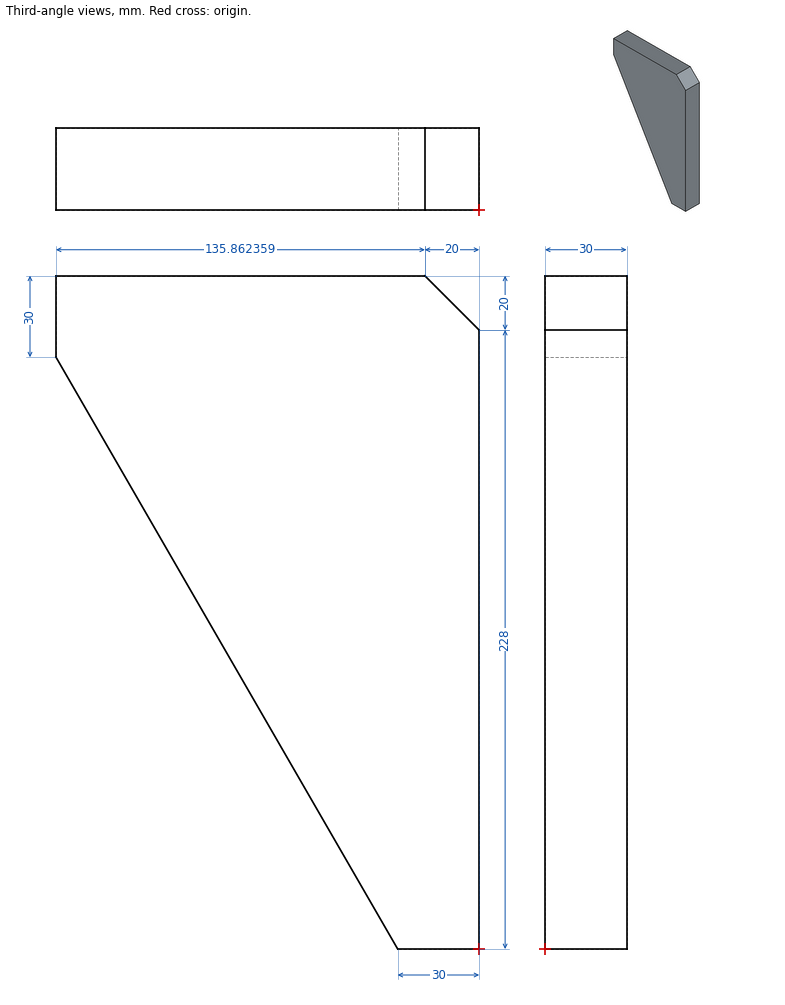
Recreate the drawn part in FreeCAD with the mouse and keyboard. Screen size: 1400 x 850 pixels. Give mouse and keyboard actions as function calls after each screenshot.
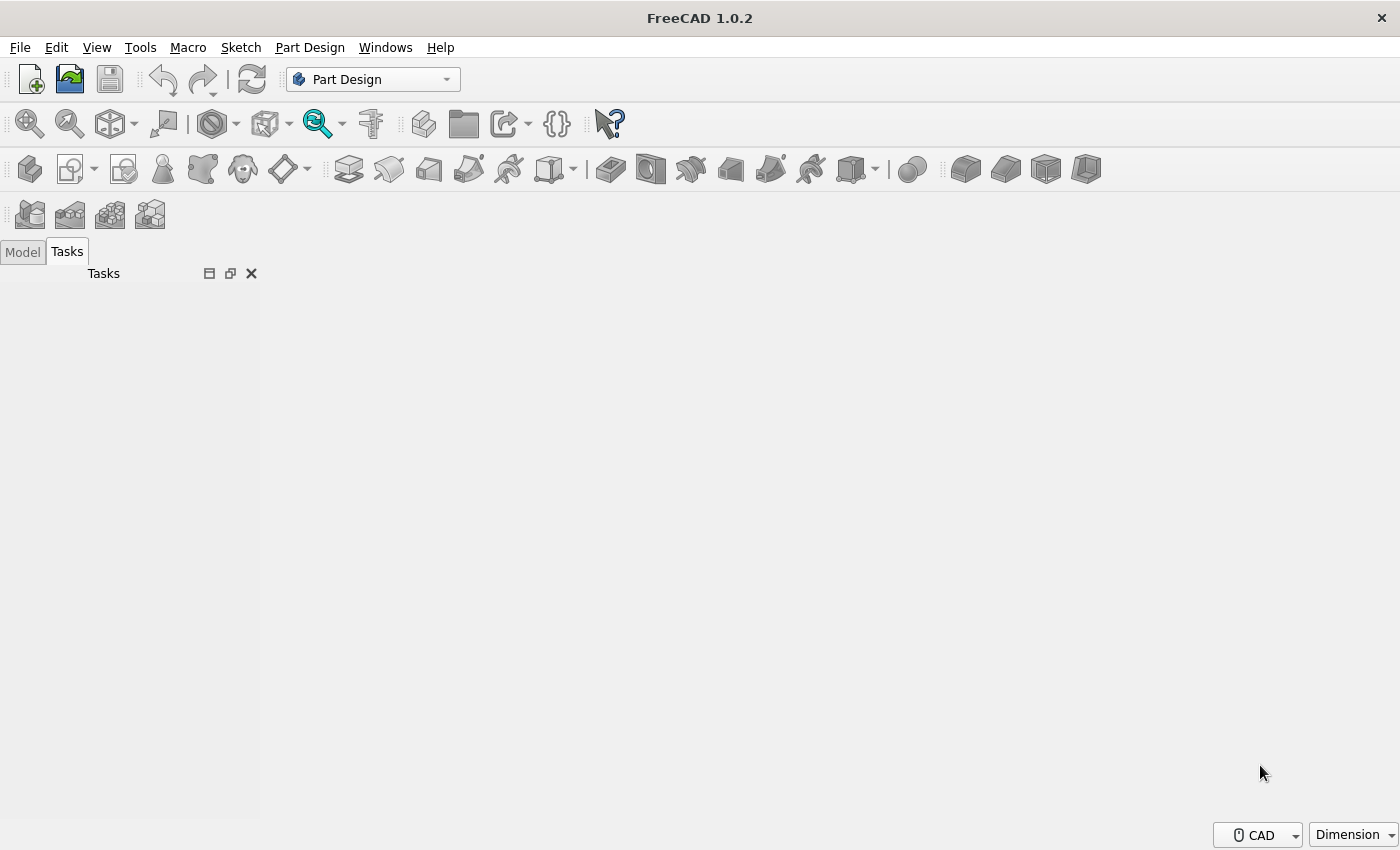
key(ctrl+n)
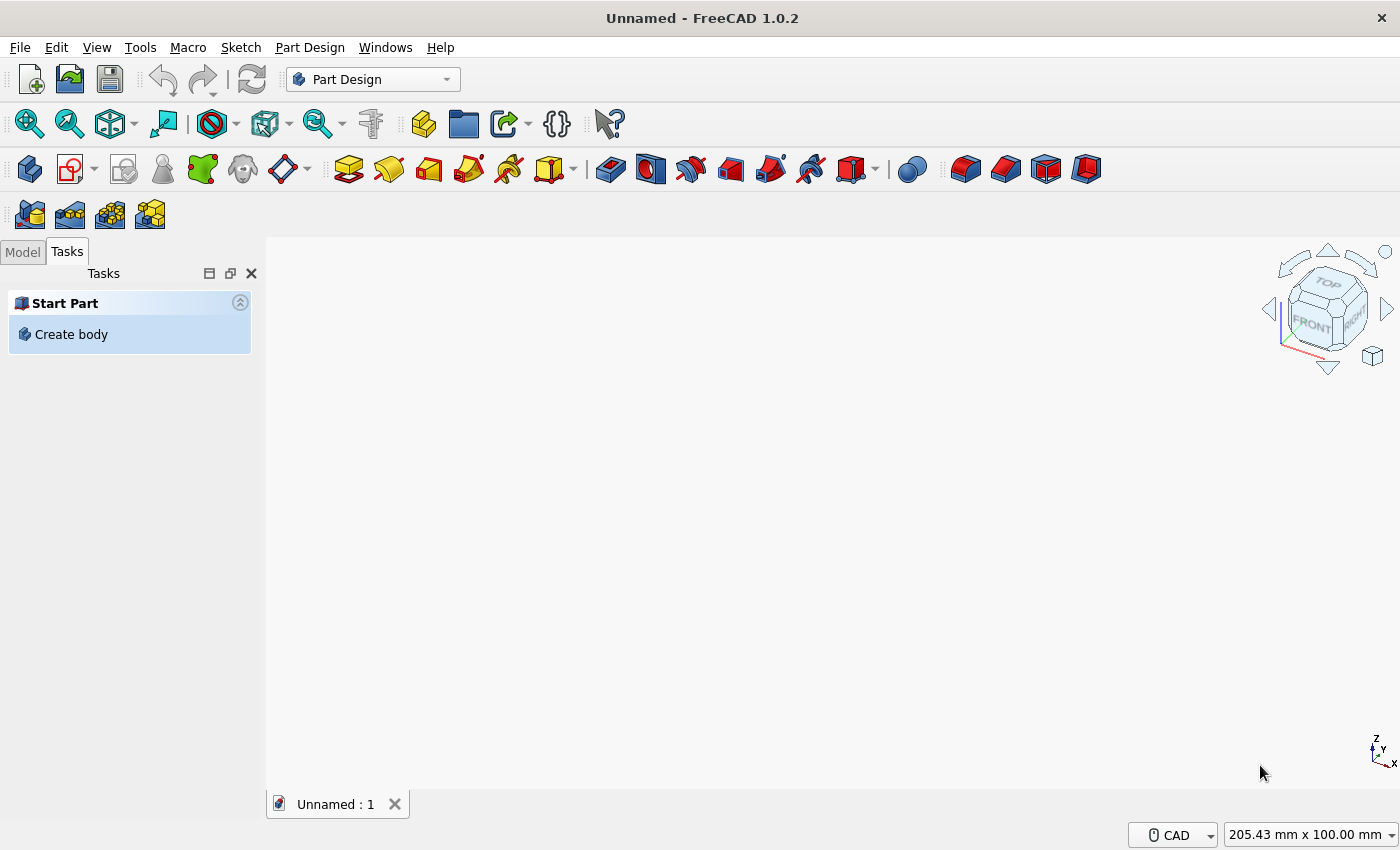
click(70, 170)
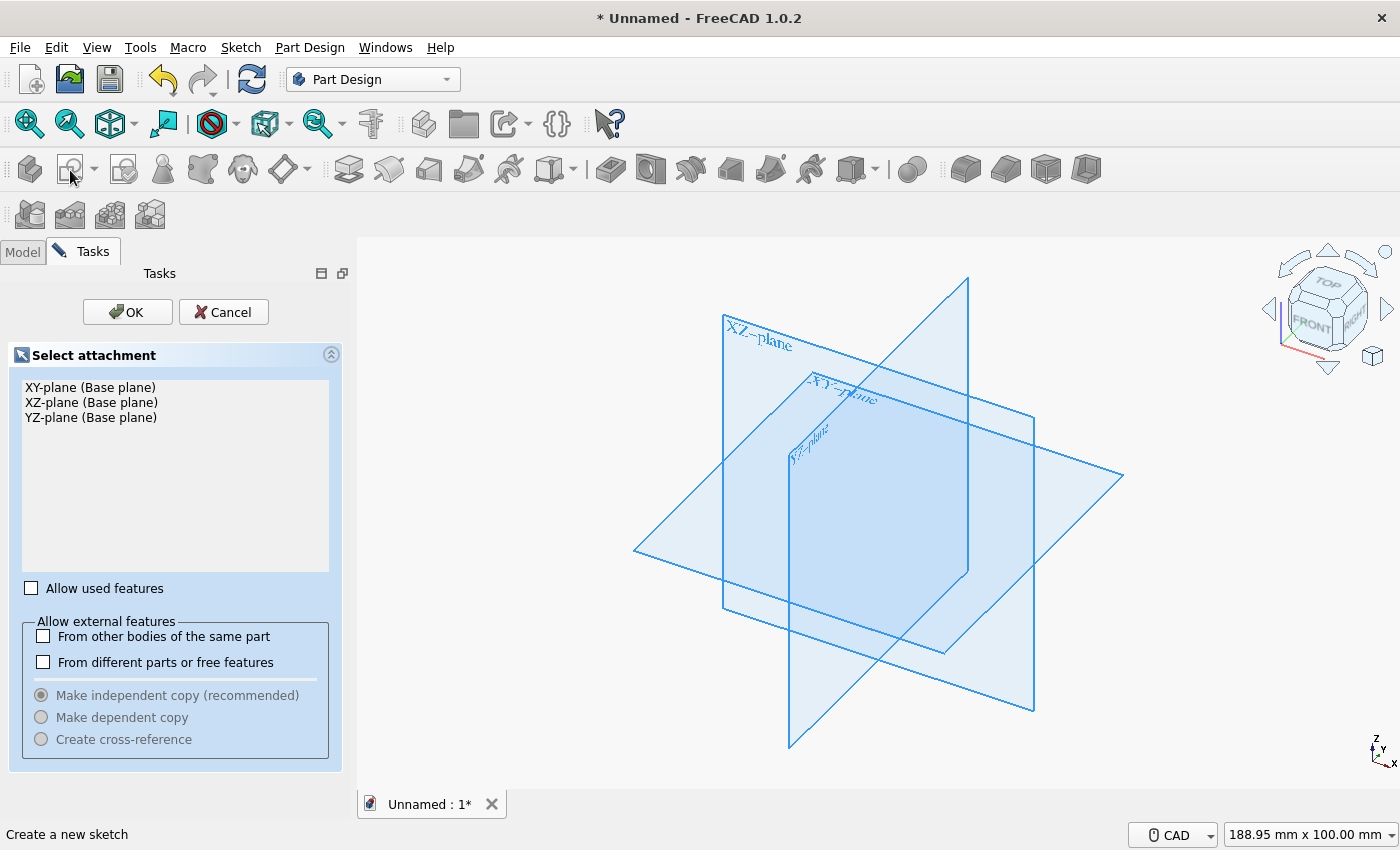
click(82, 402)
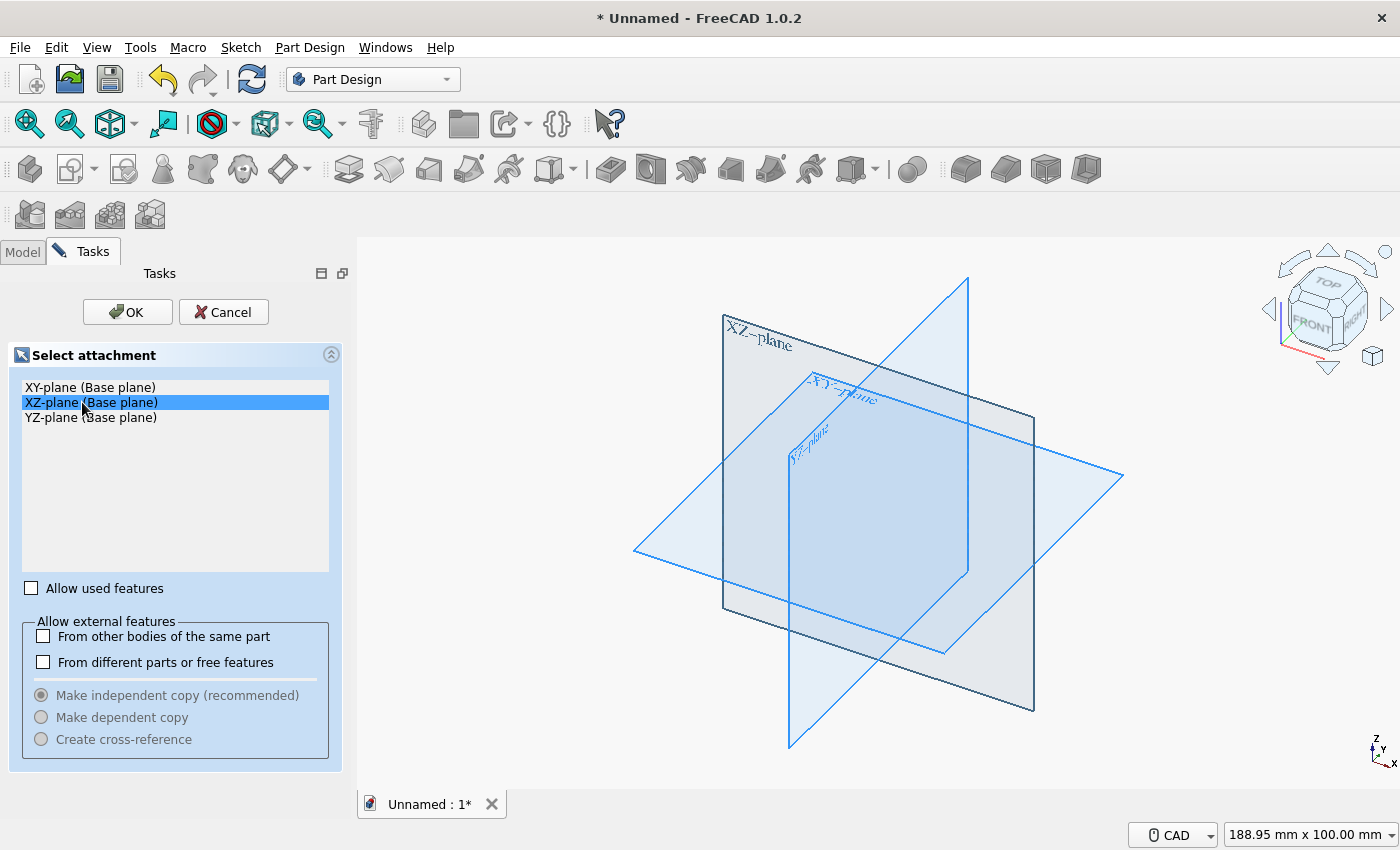
click(128, 312)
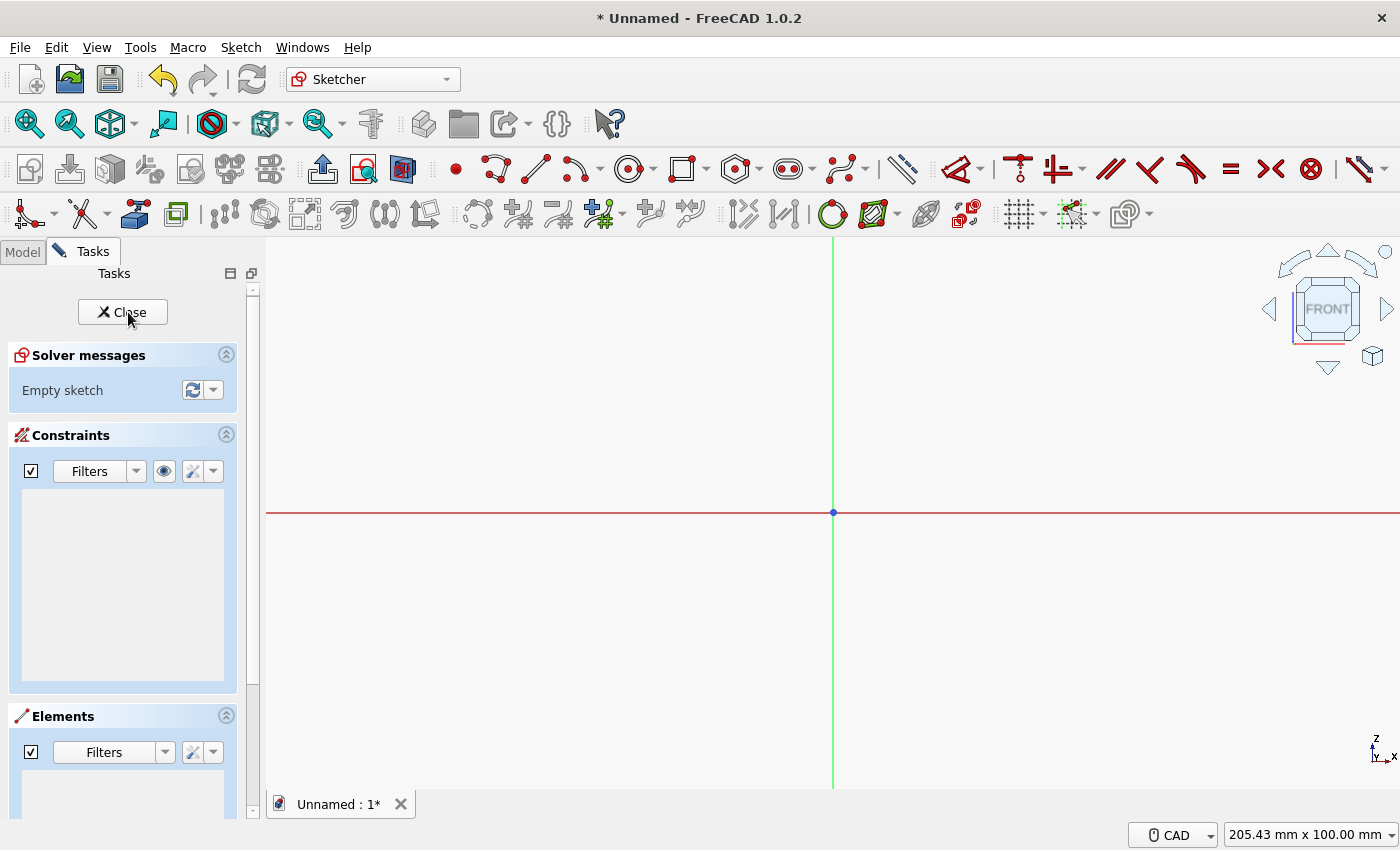
scroll(883, 737, down, 7)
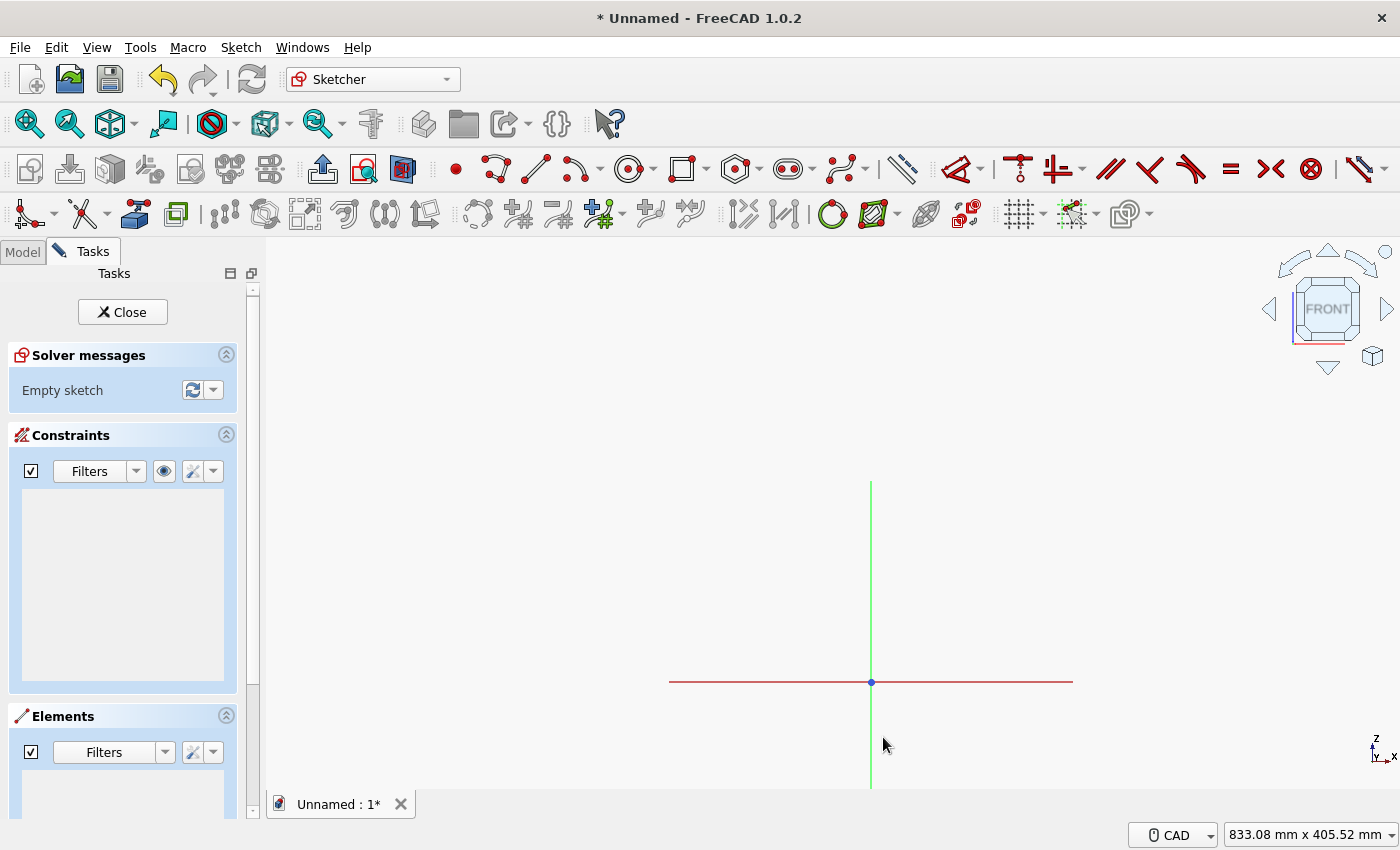
key(g)
key(m)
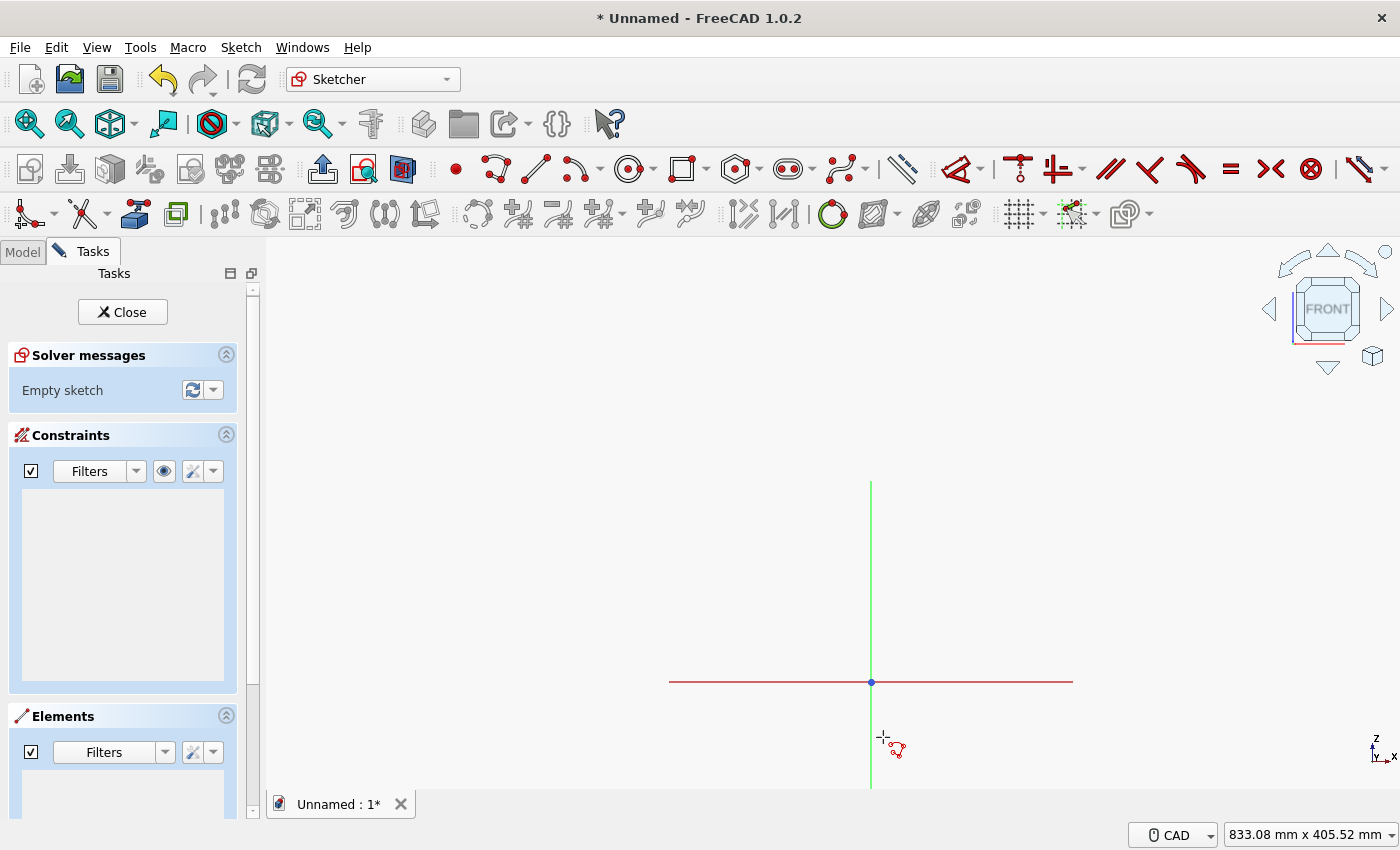
click(871, 682)
click(830, 673)
click(659, 386)
click(659, 345)
click(844, 345)
click(862, 372)
click(871, 682)
key(Escape)
key(Escape)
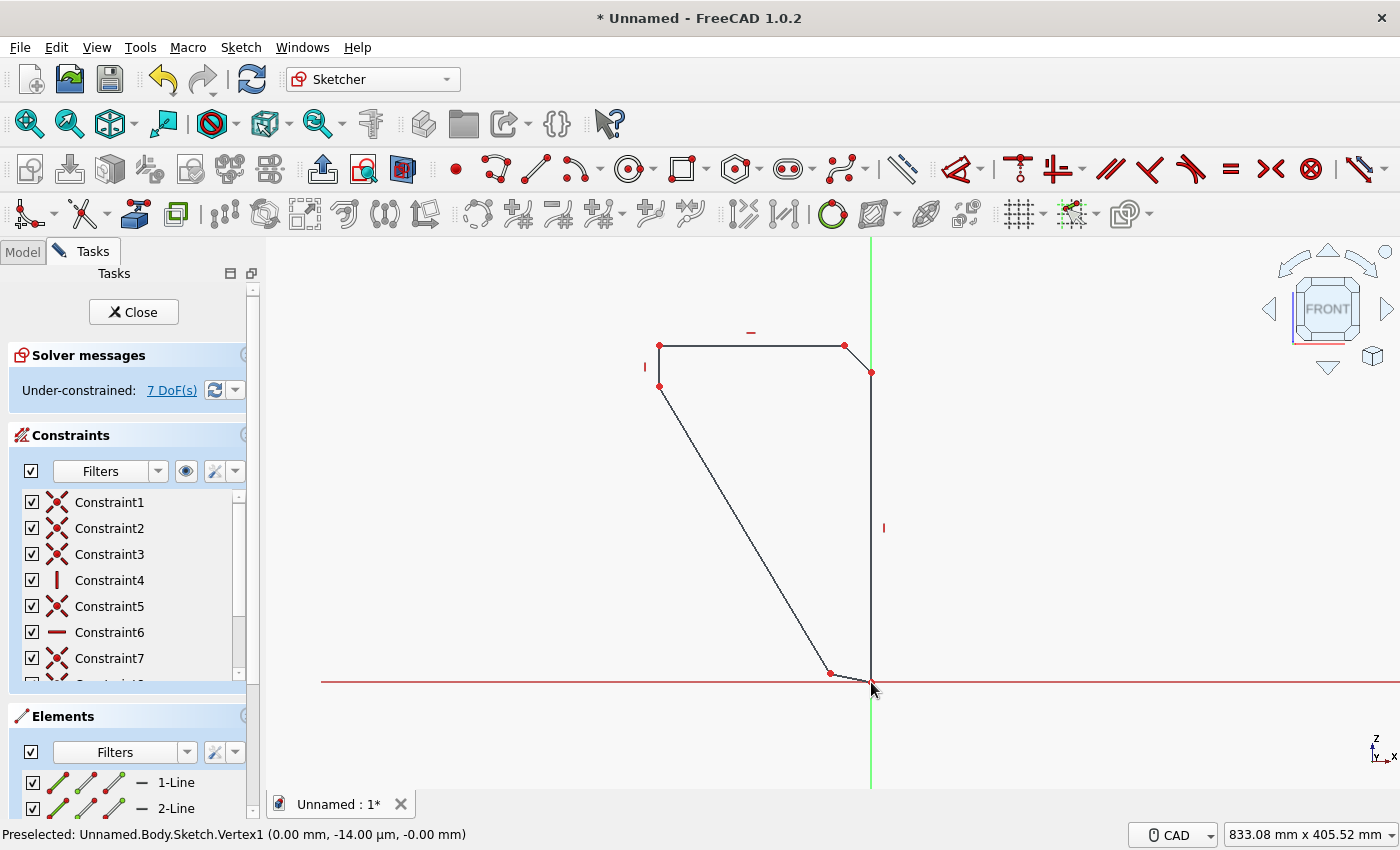
click(859, 680)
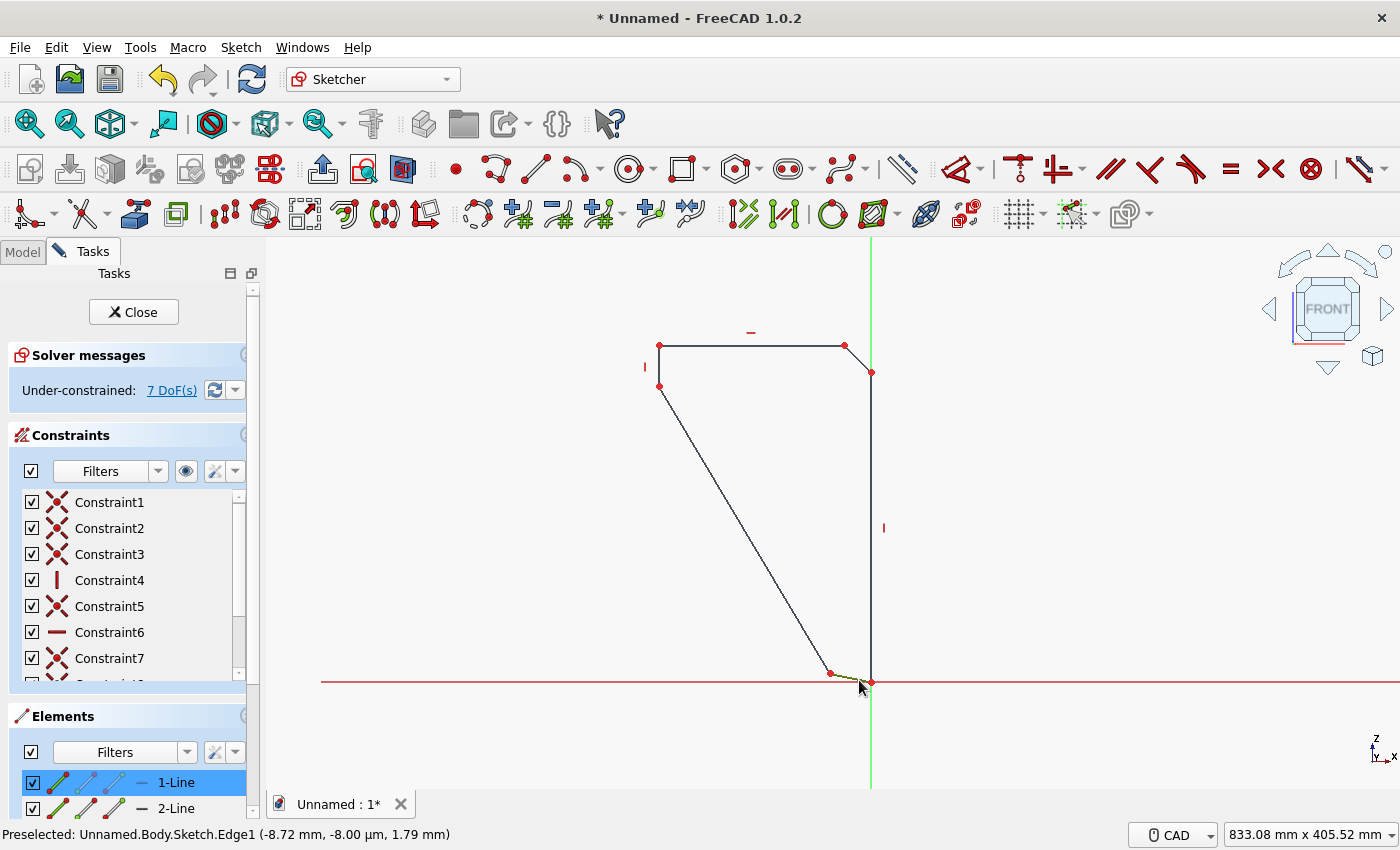
key(h)